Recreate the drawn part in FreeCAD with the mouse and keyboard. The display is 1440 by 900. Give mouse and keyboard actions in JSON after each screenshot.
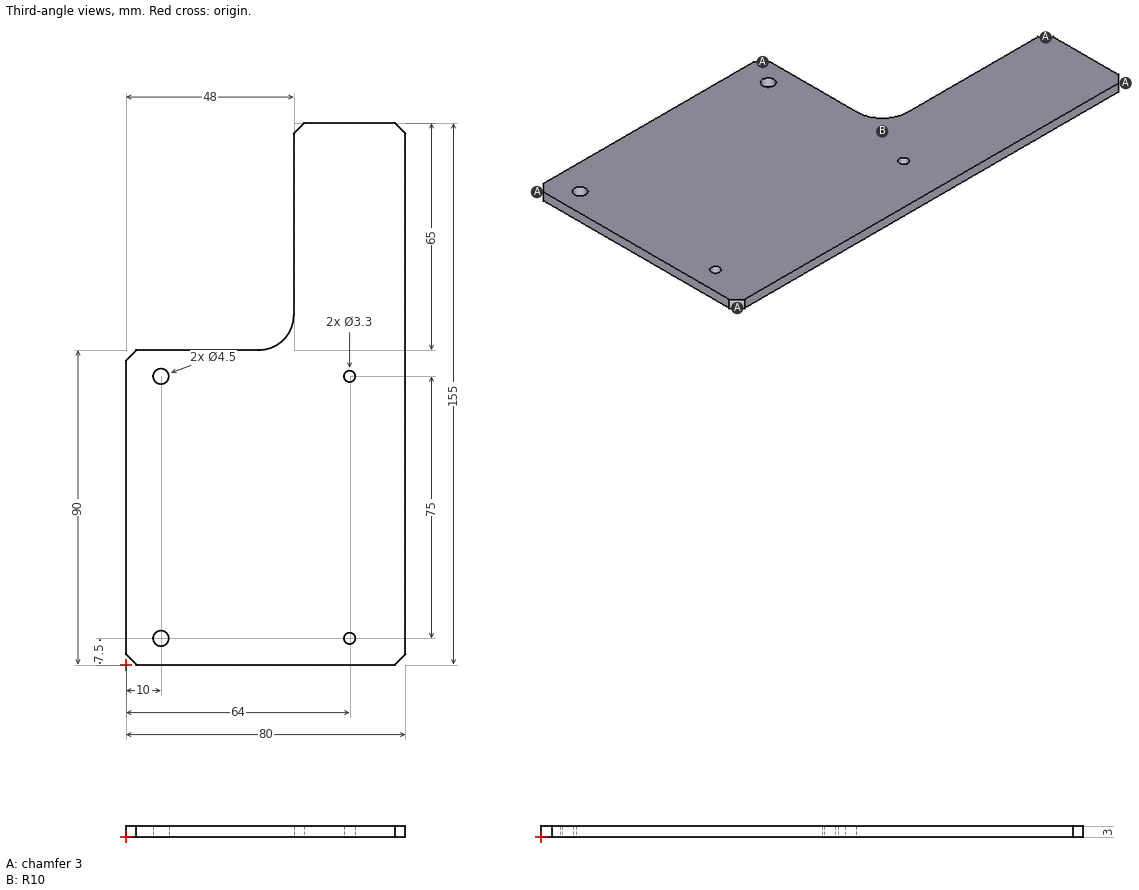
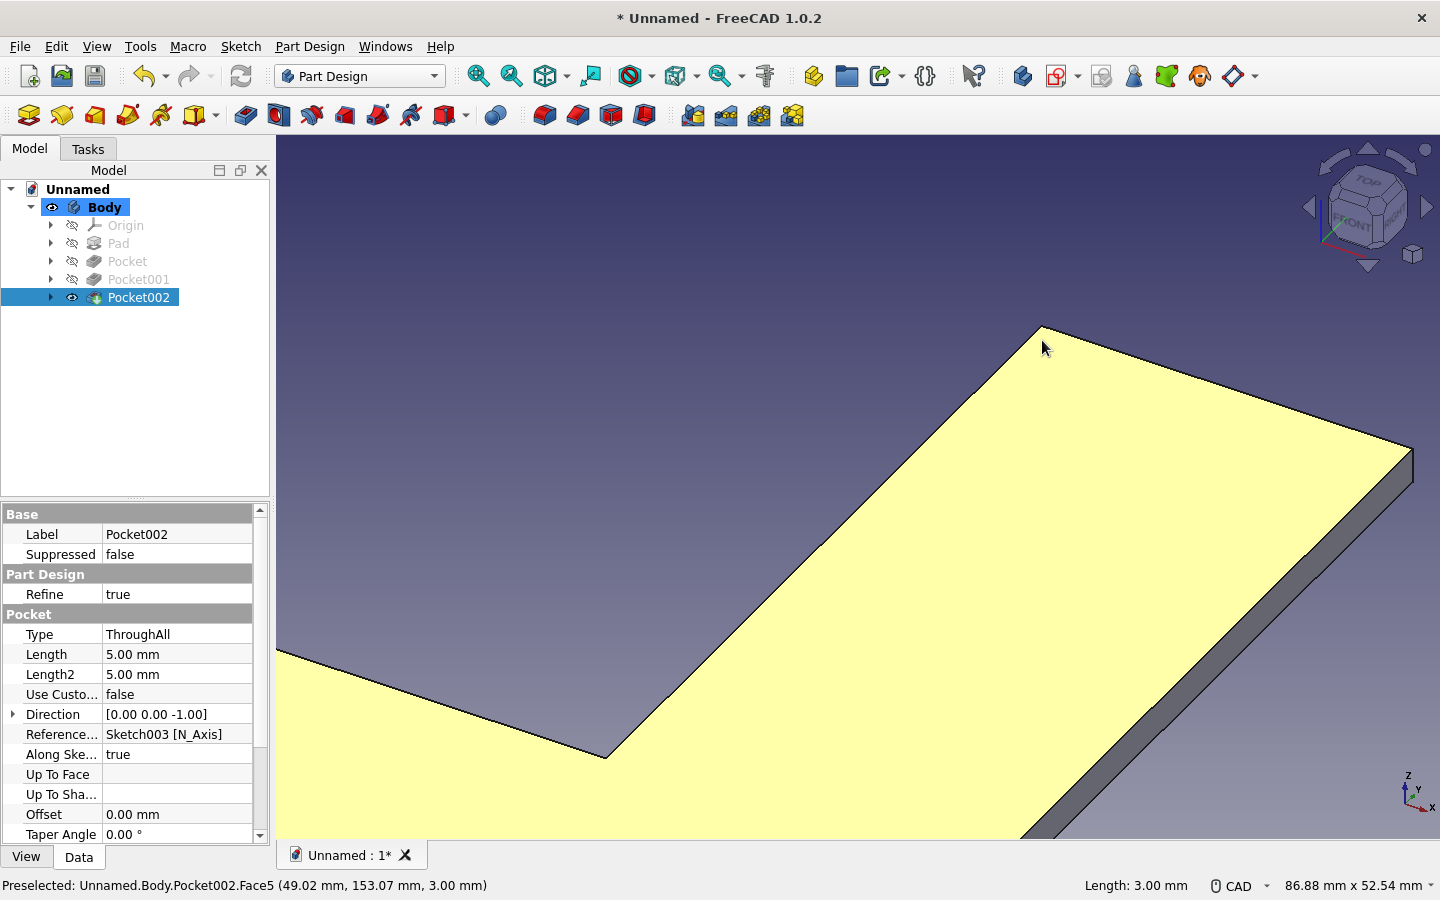
{"action": "key", "text": "v f"}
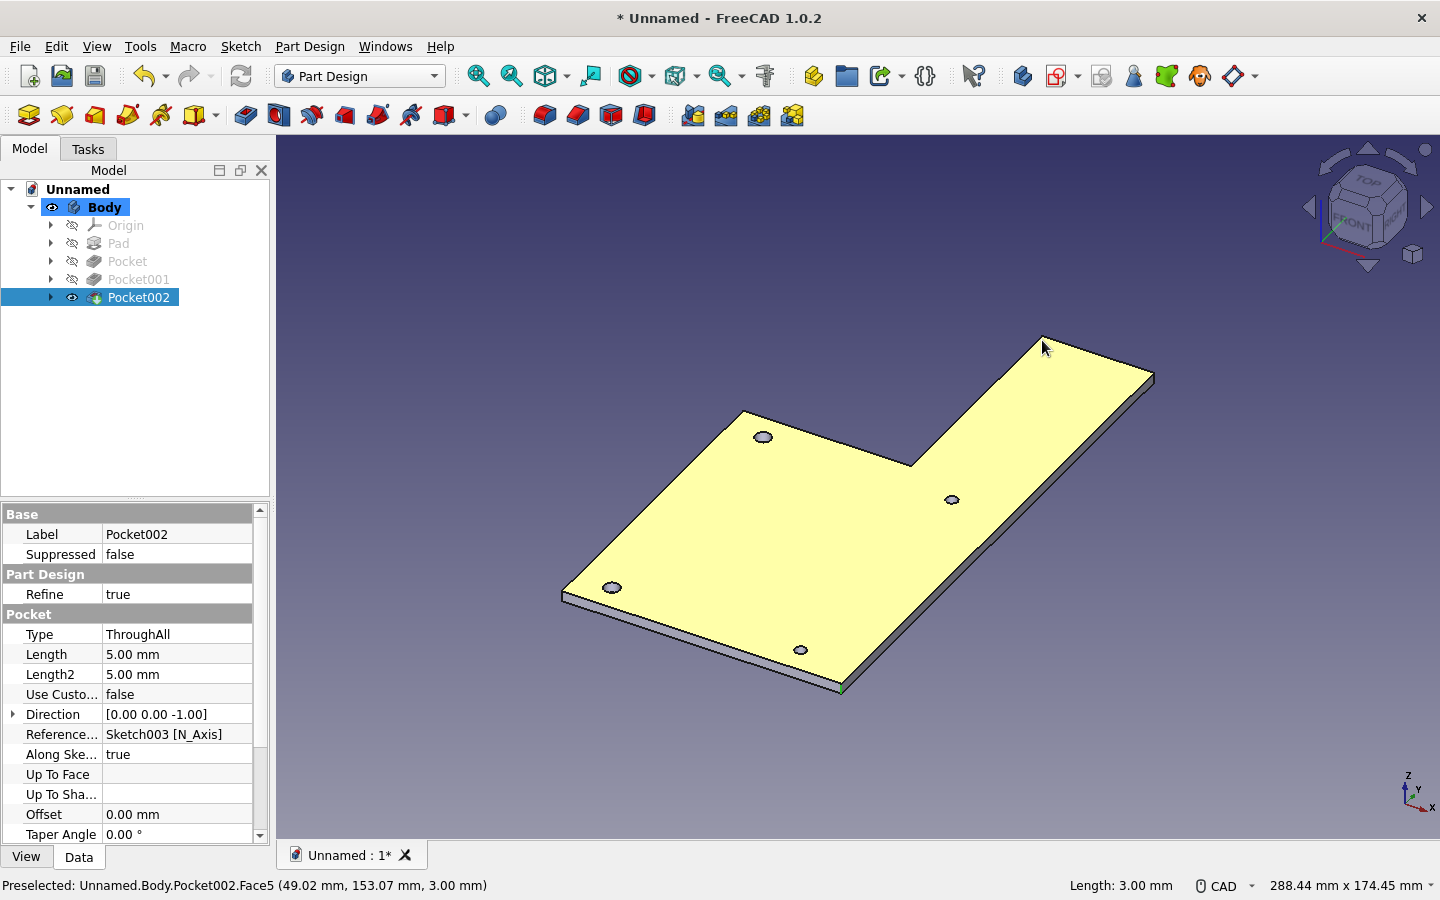
{"action": "key", "text": "0"}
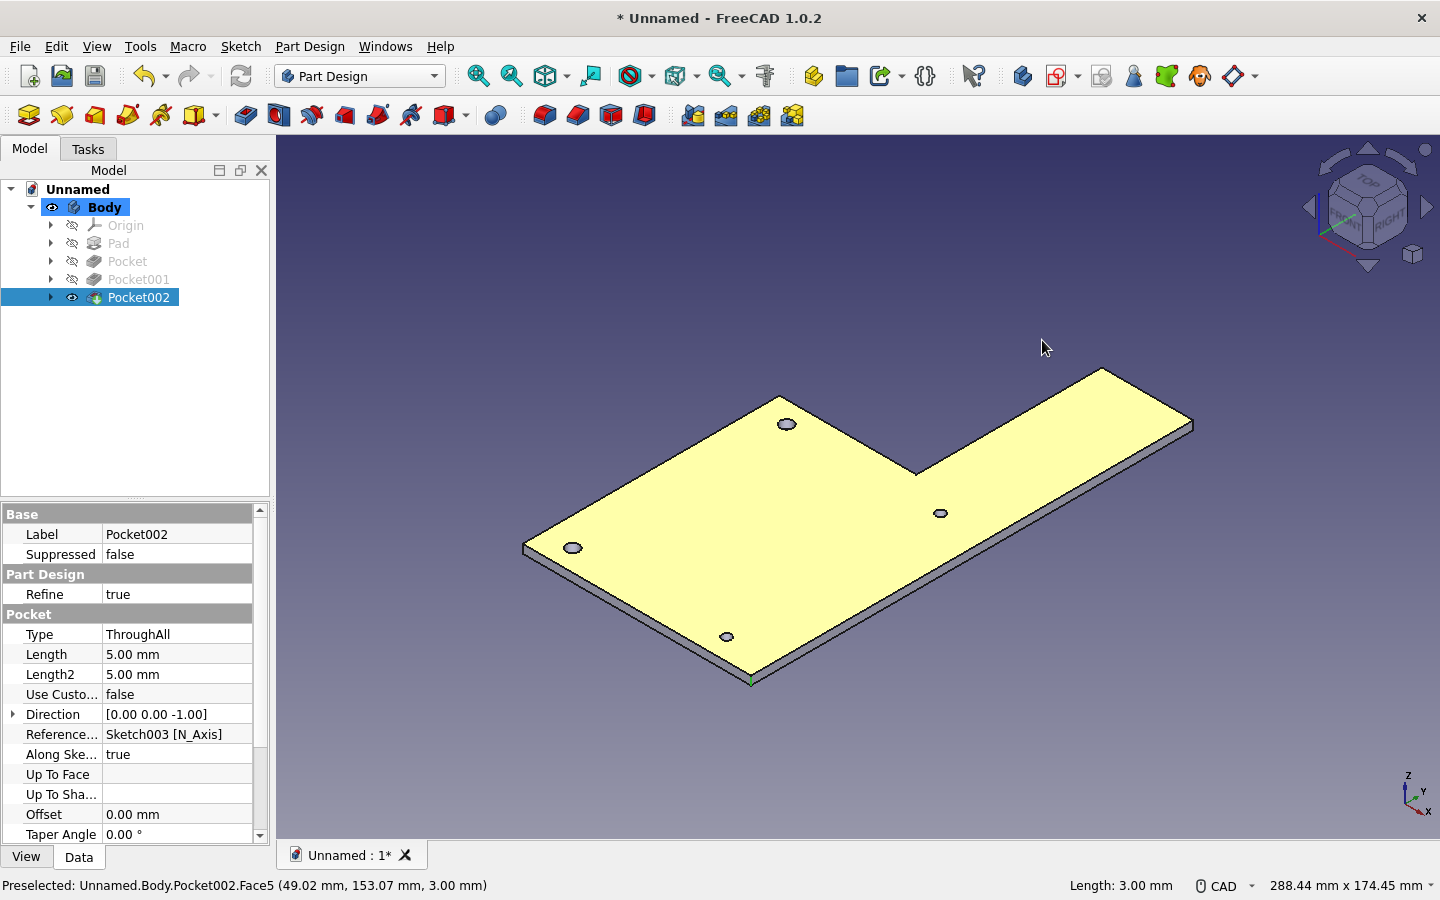
{"action": "scroll", "coordinate": [1102, 372], "scroll_direction": "up", "scroll_amount": 6}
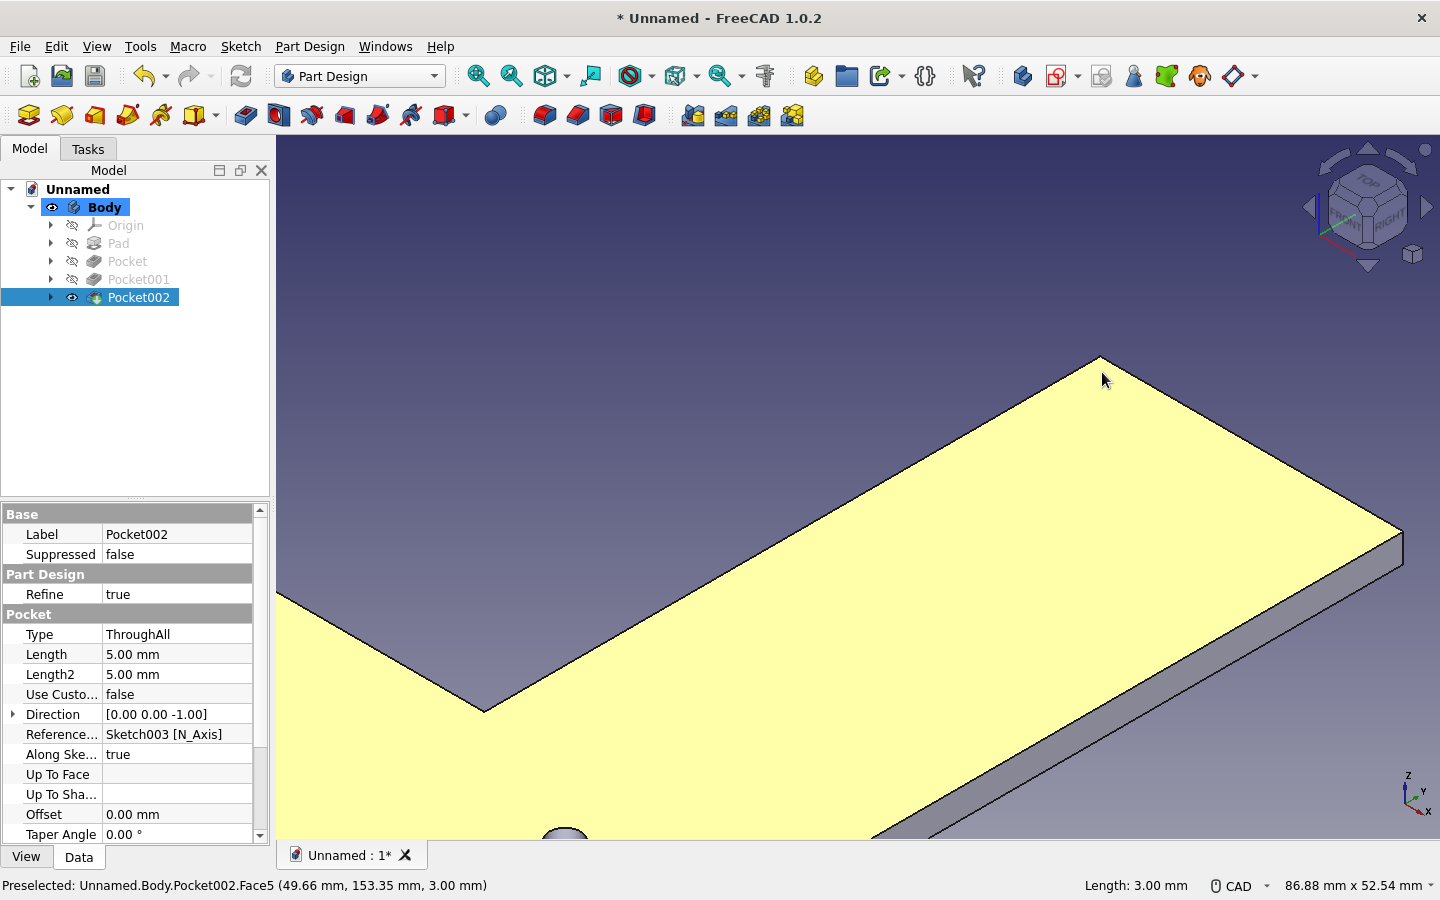
{"action": "key", "text": "v f"}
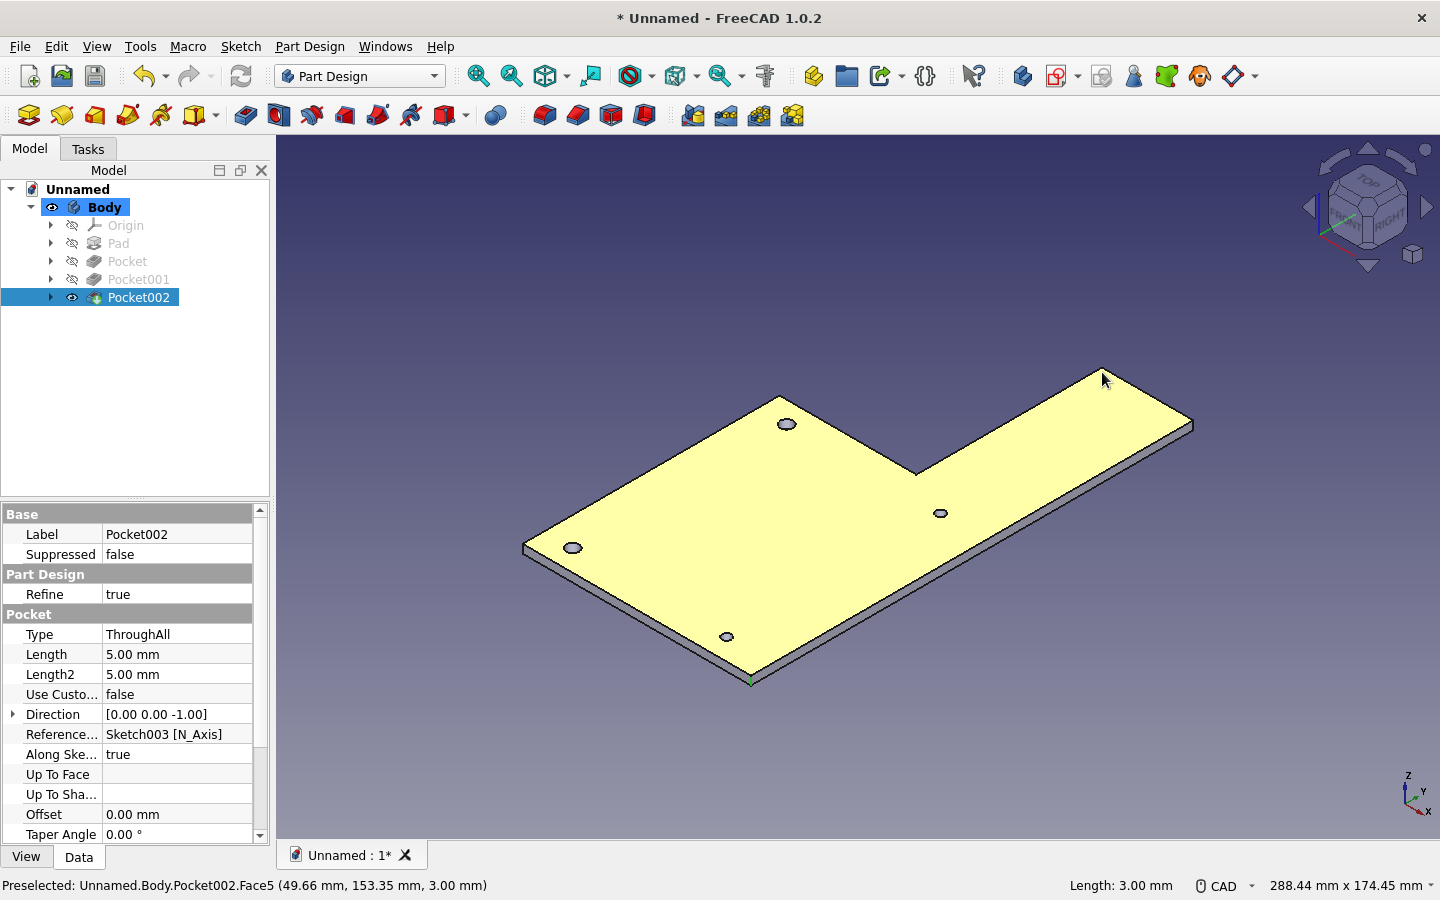
{"action": "key", "text": "2"}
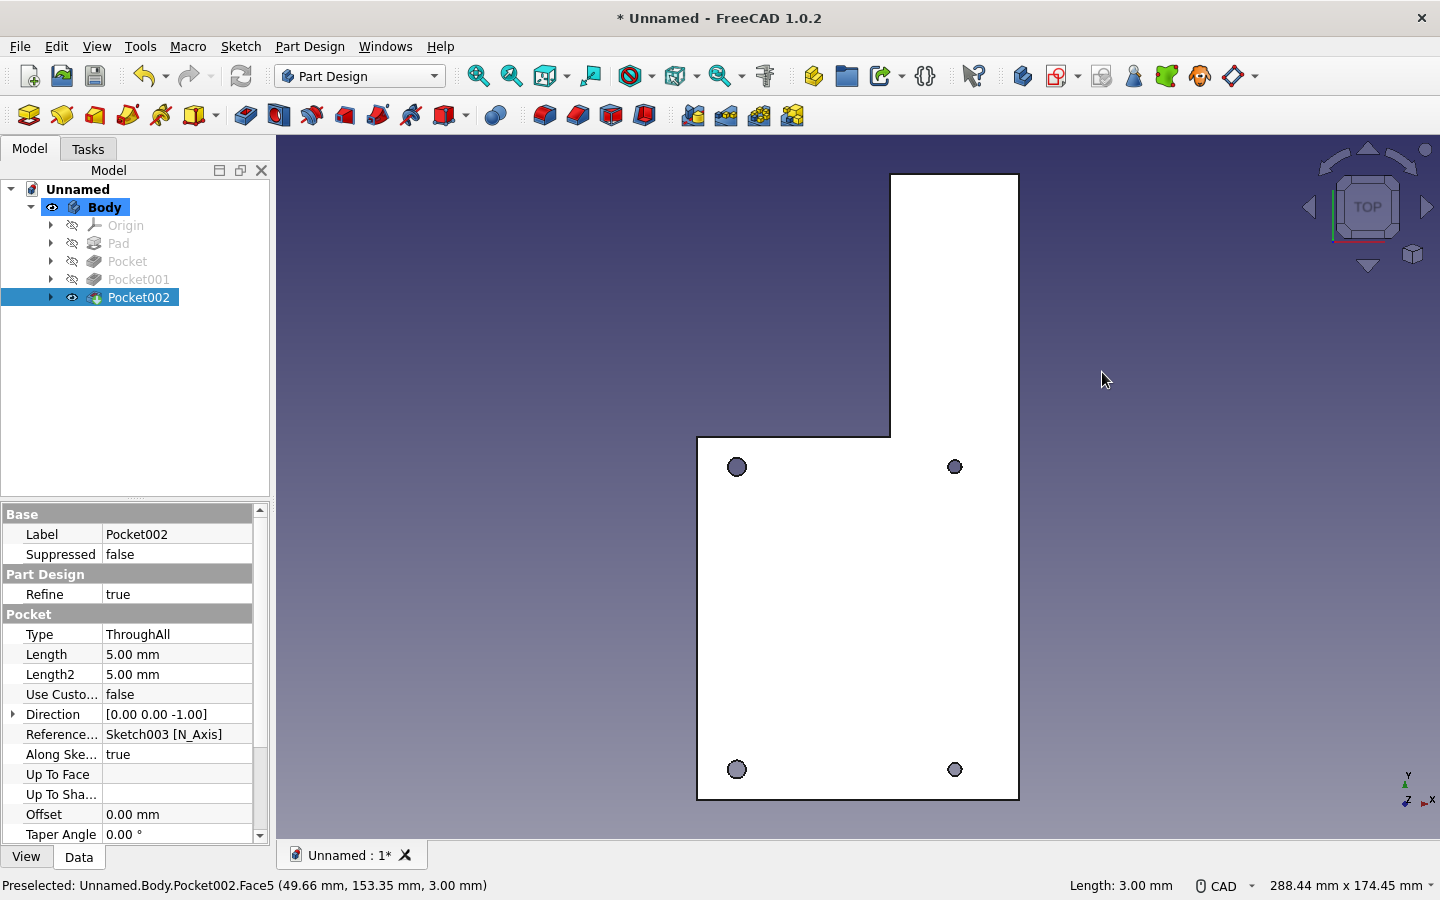
{"action": "scroll", "coordinate": [890, 173], "scroll_direction": "up", "scroll_amount": 6}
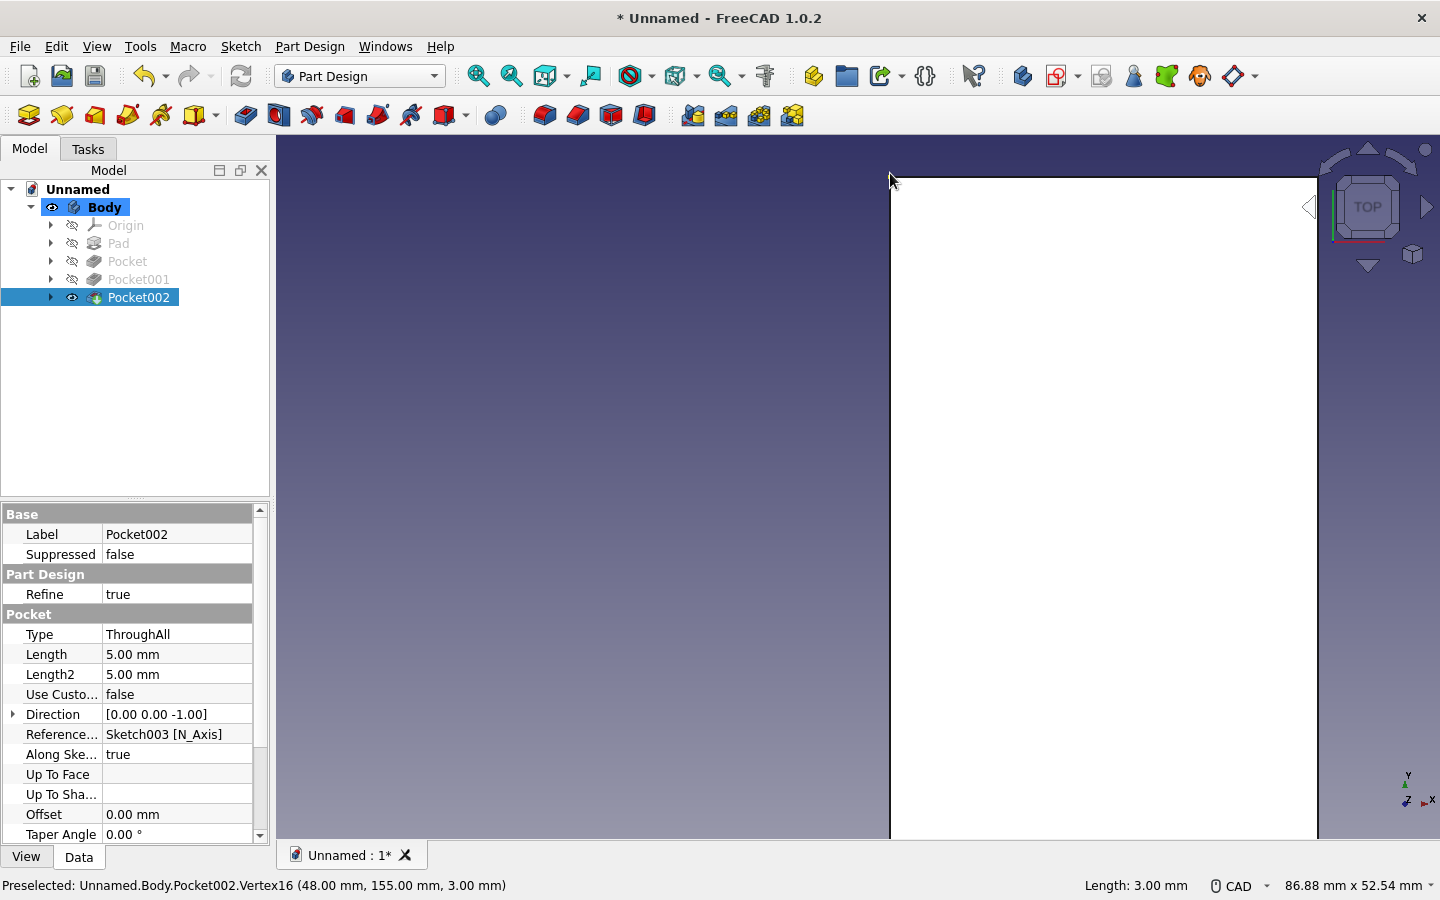
{"action": "key", "text": "v f"}